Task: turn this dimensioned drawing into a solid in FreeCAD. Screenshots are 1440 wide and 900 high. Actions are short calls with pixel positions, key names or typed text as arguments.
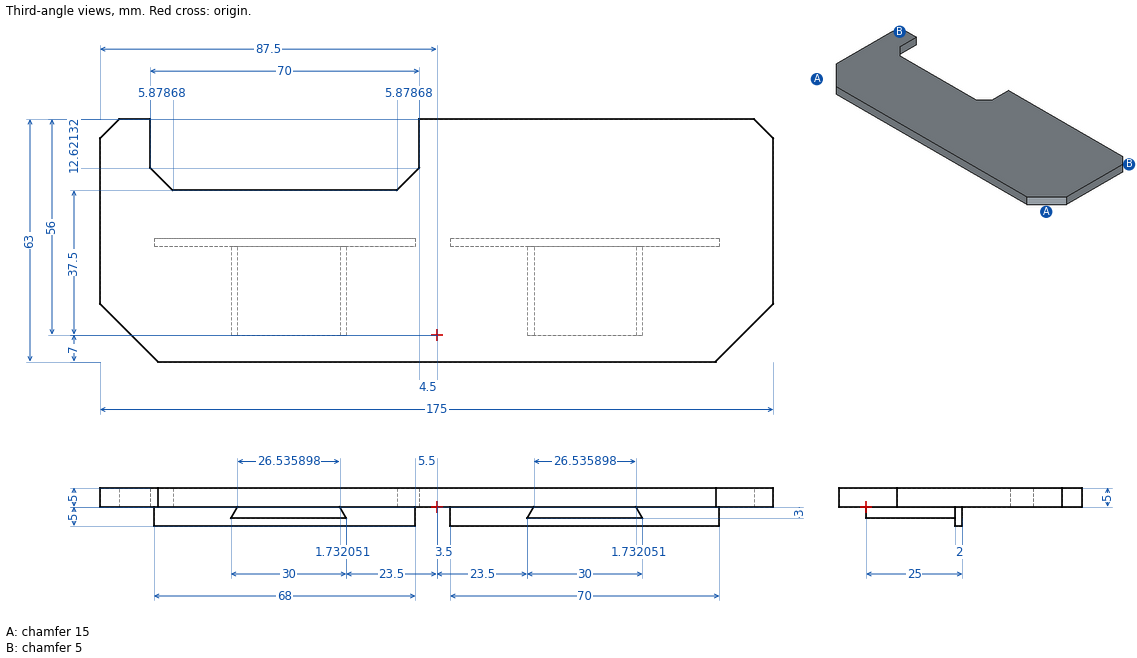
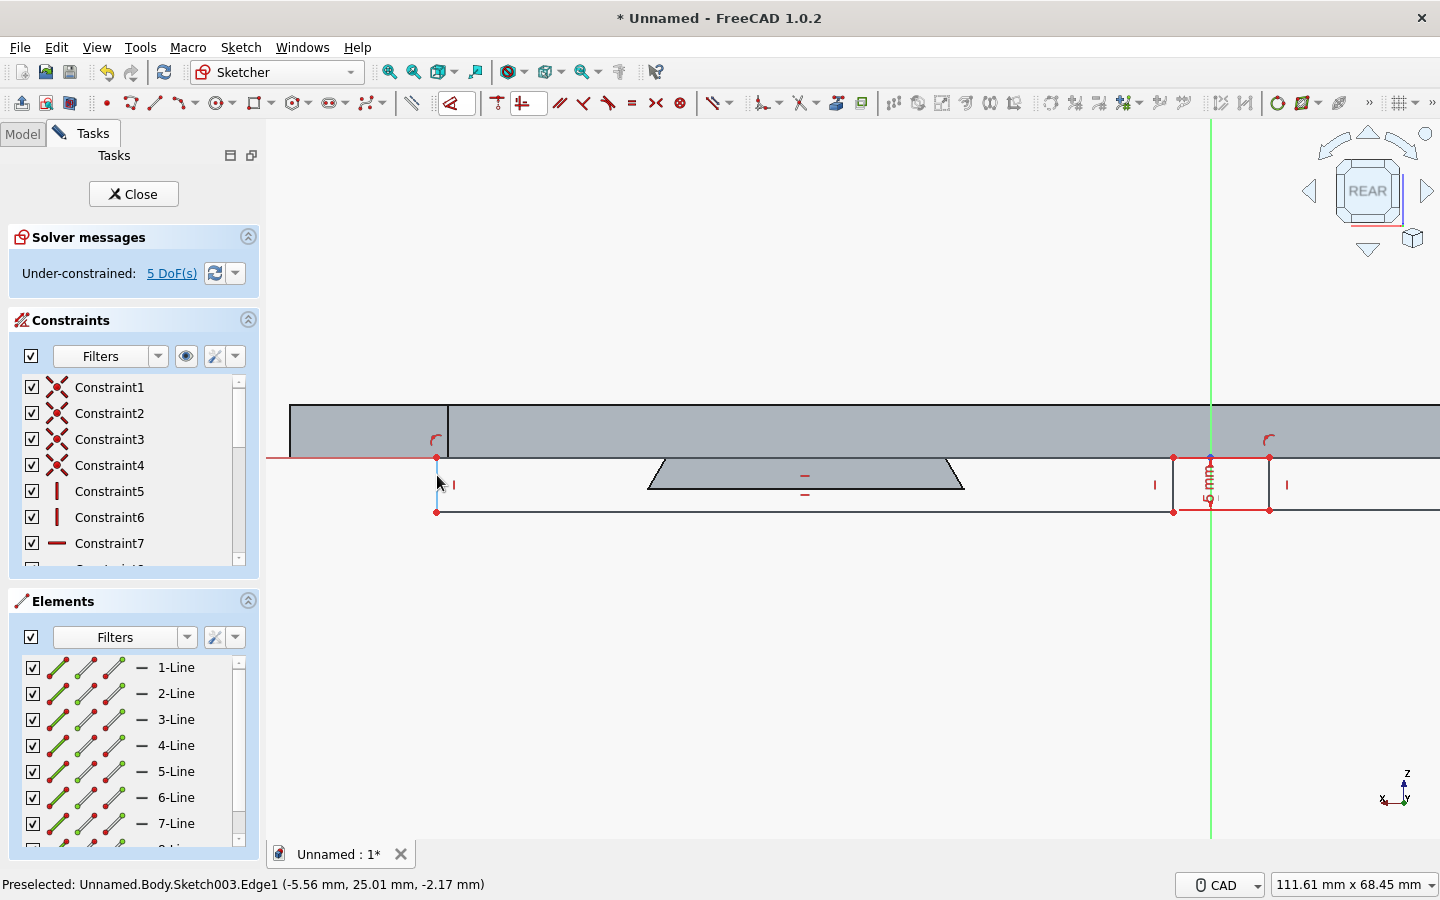
click(437, 474)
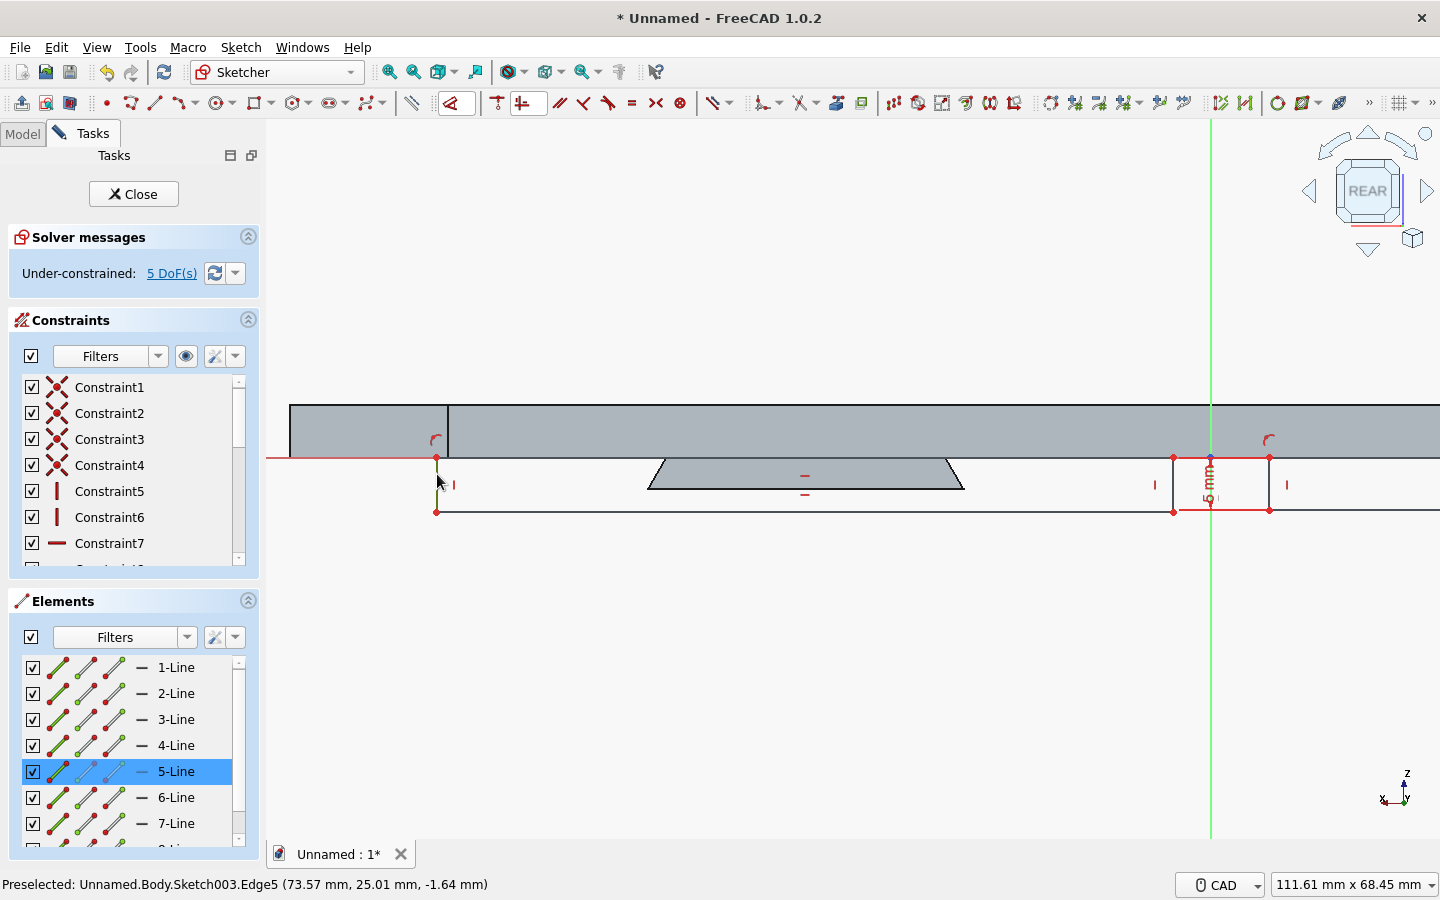
key(i)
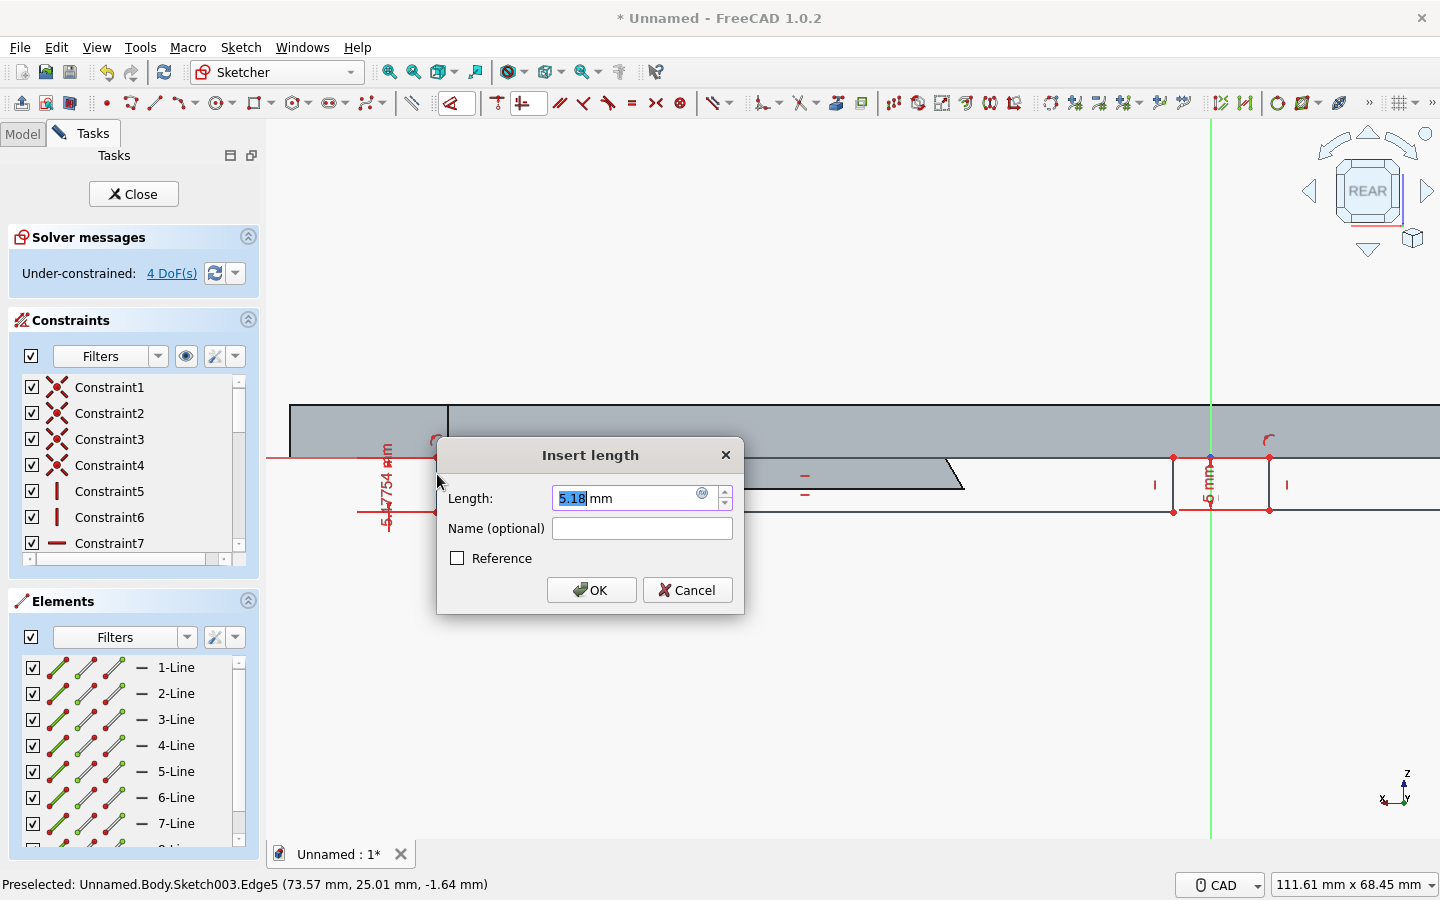
text(5)
key(Return)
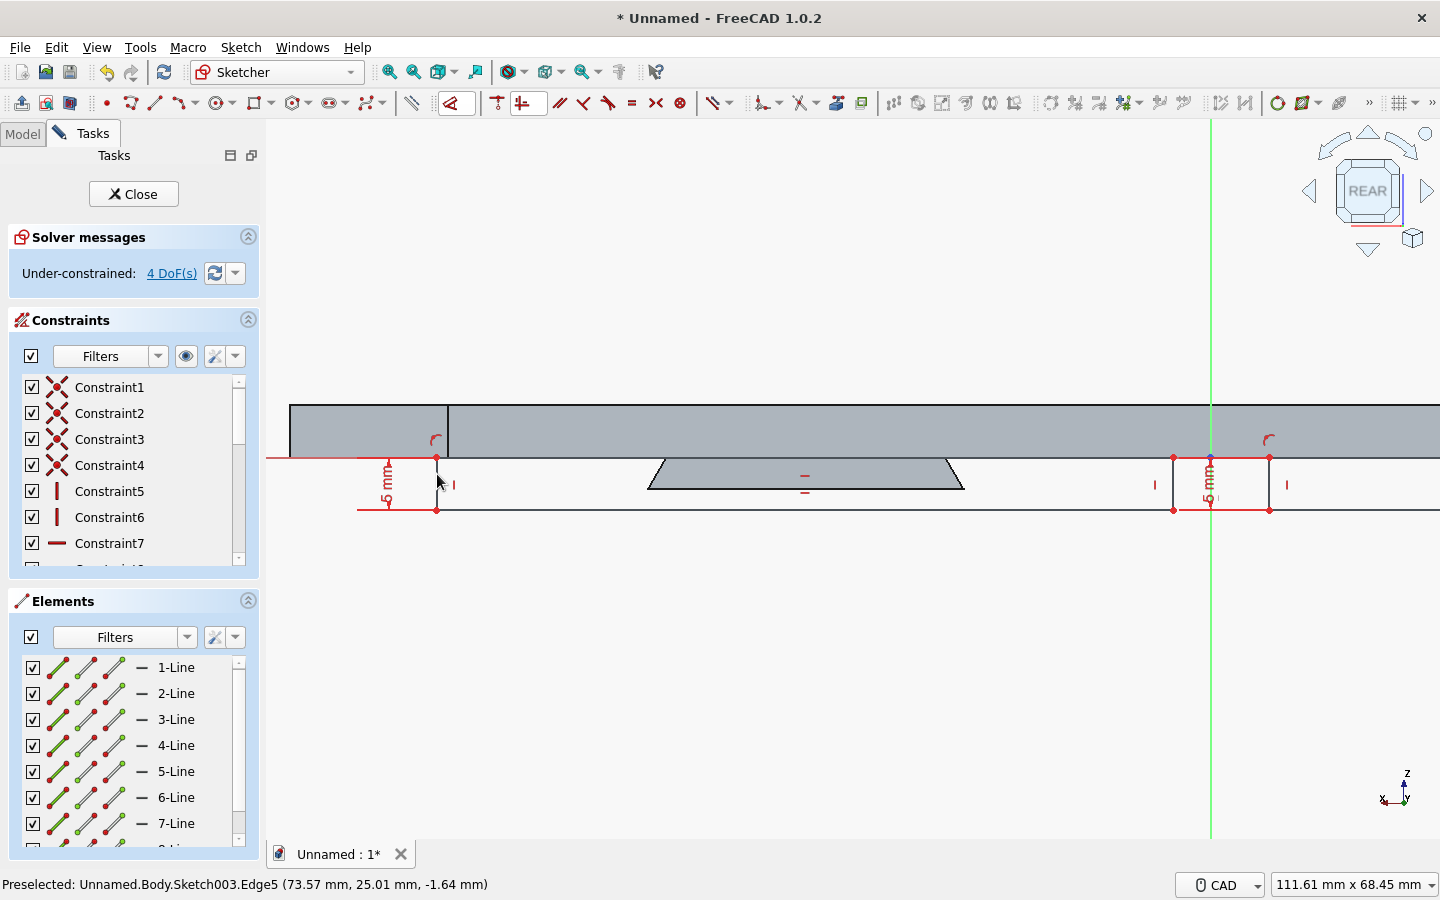
scroll(437, 475, down, 4)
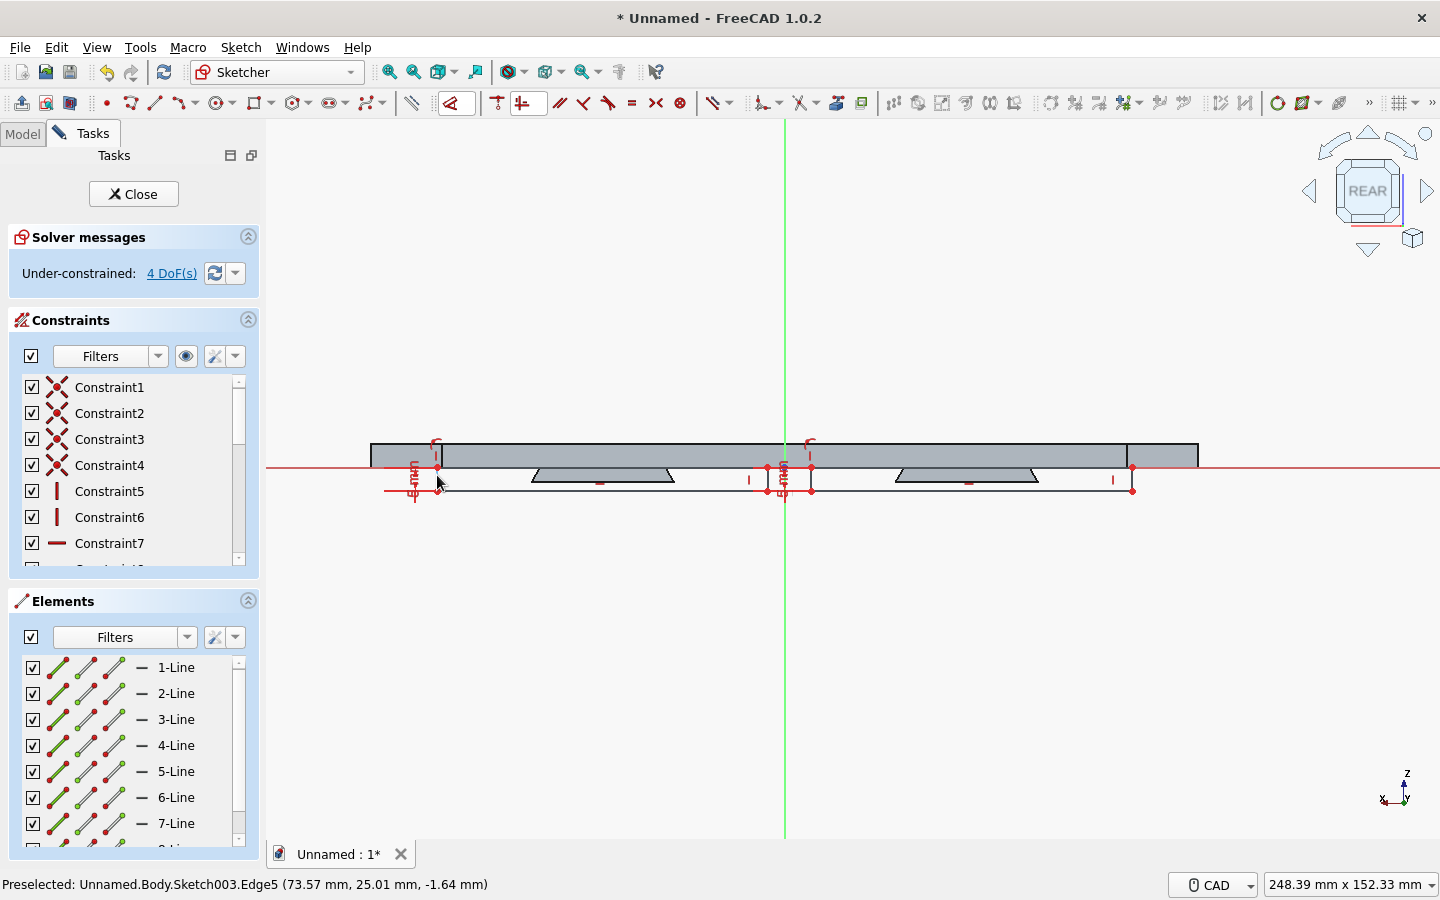
click(907, 491)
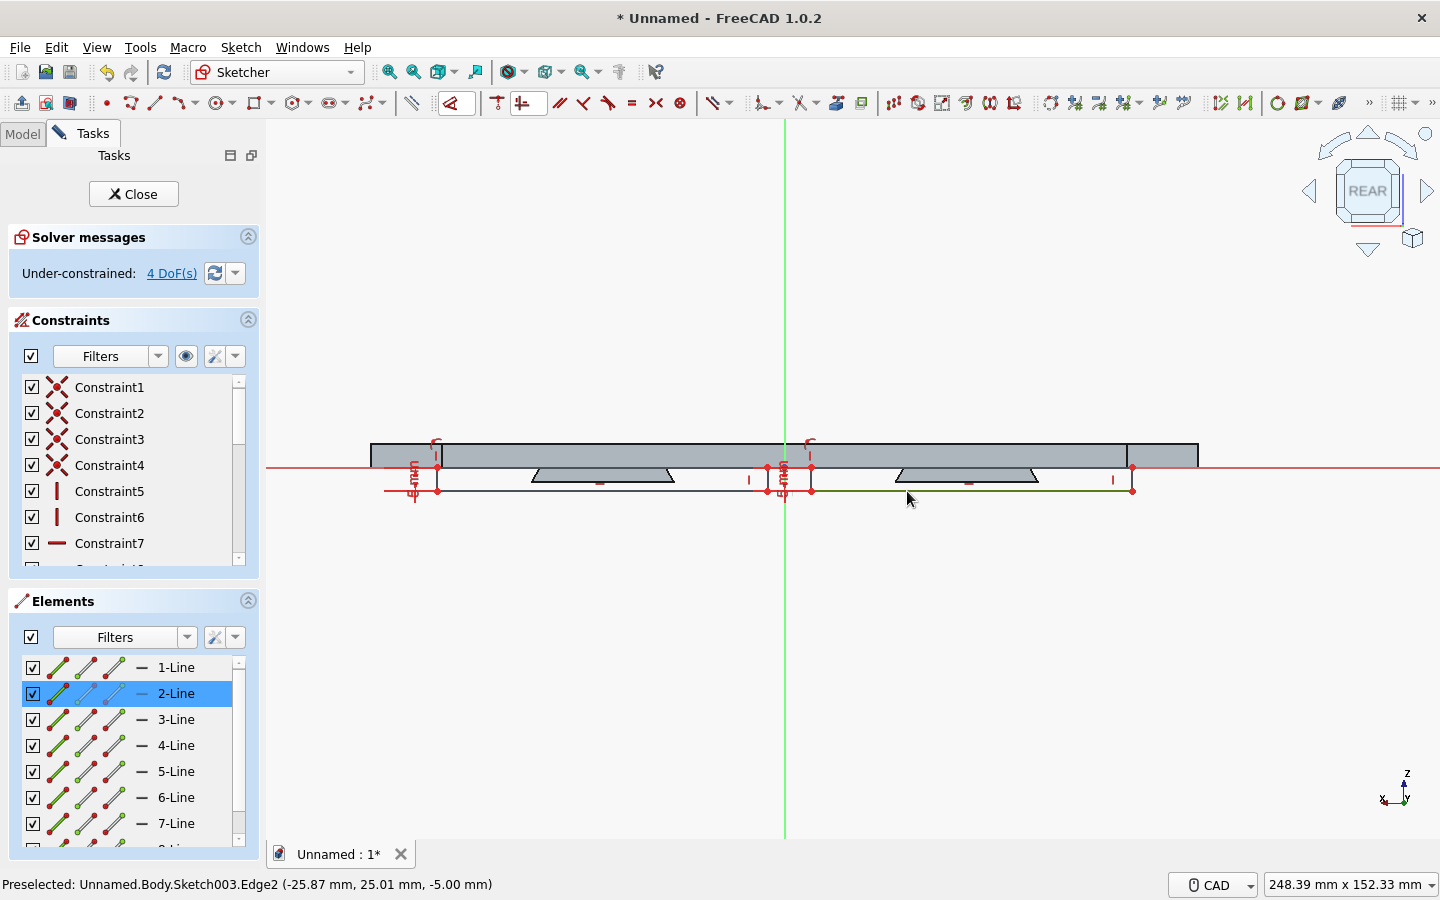
click(470, 104)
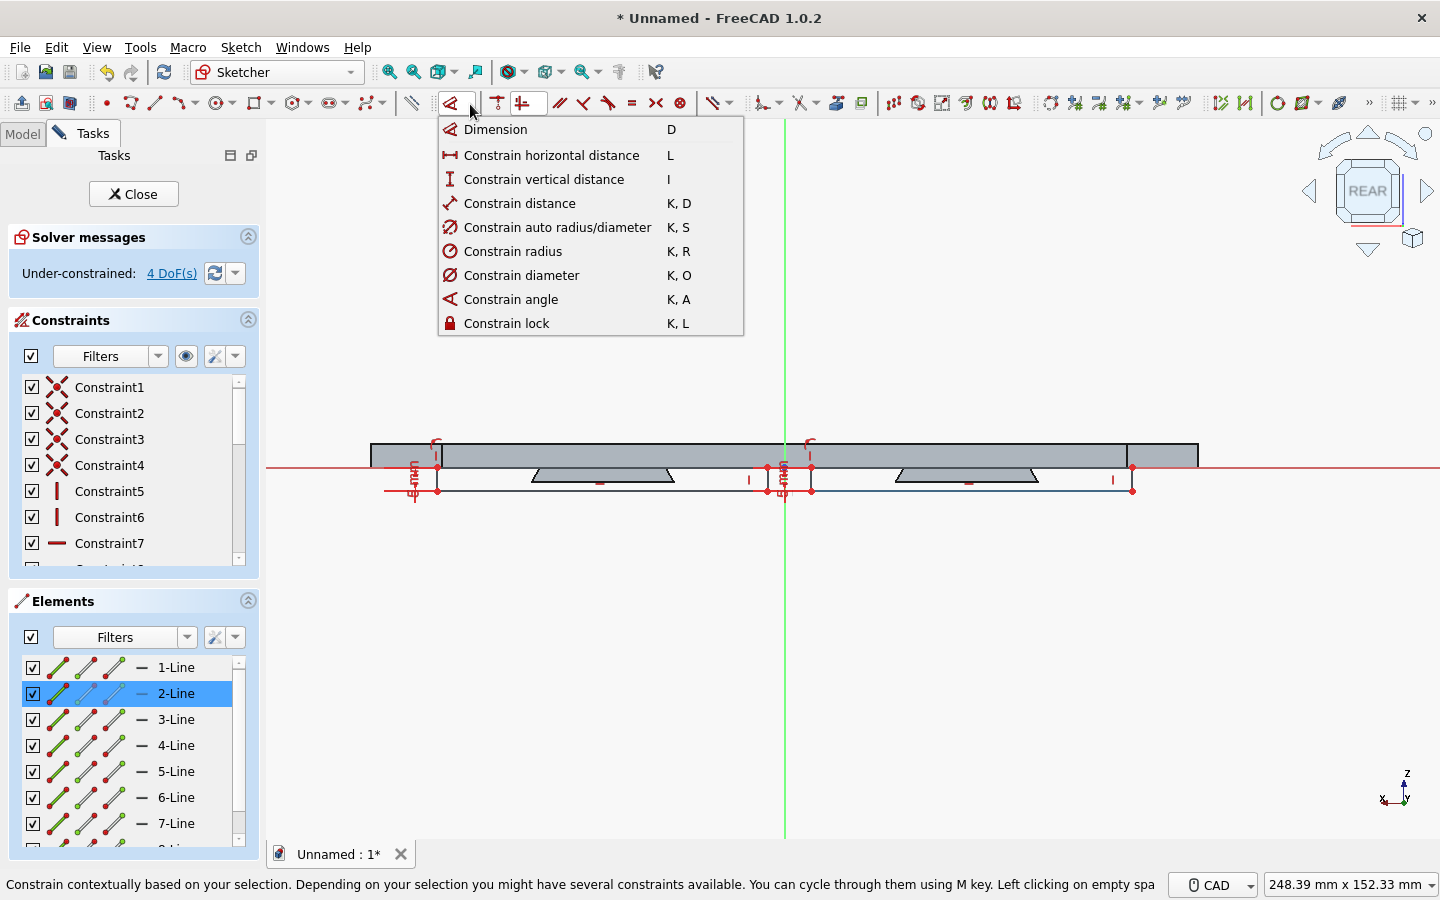
click(591, 155)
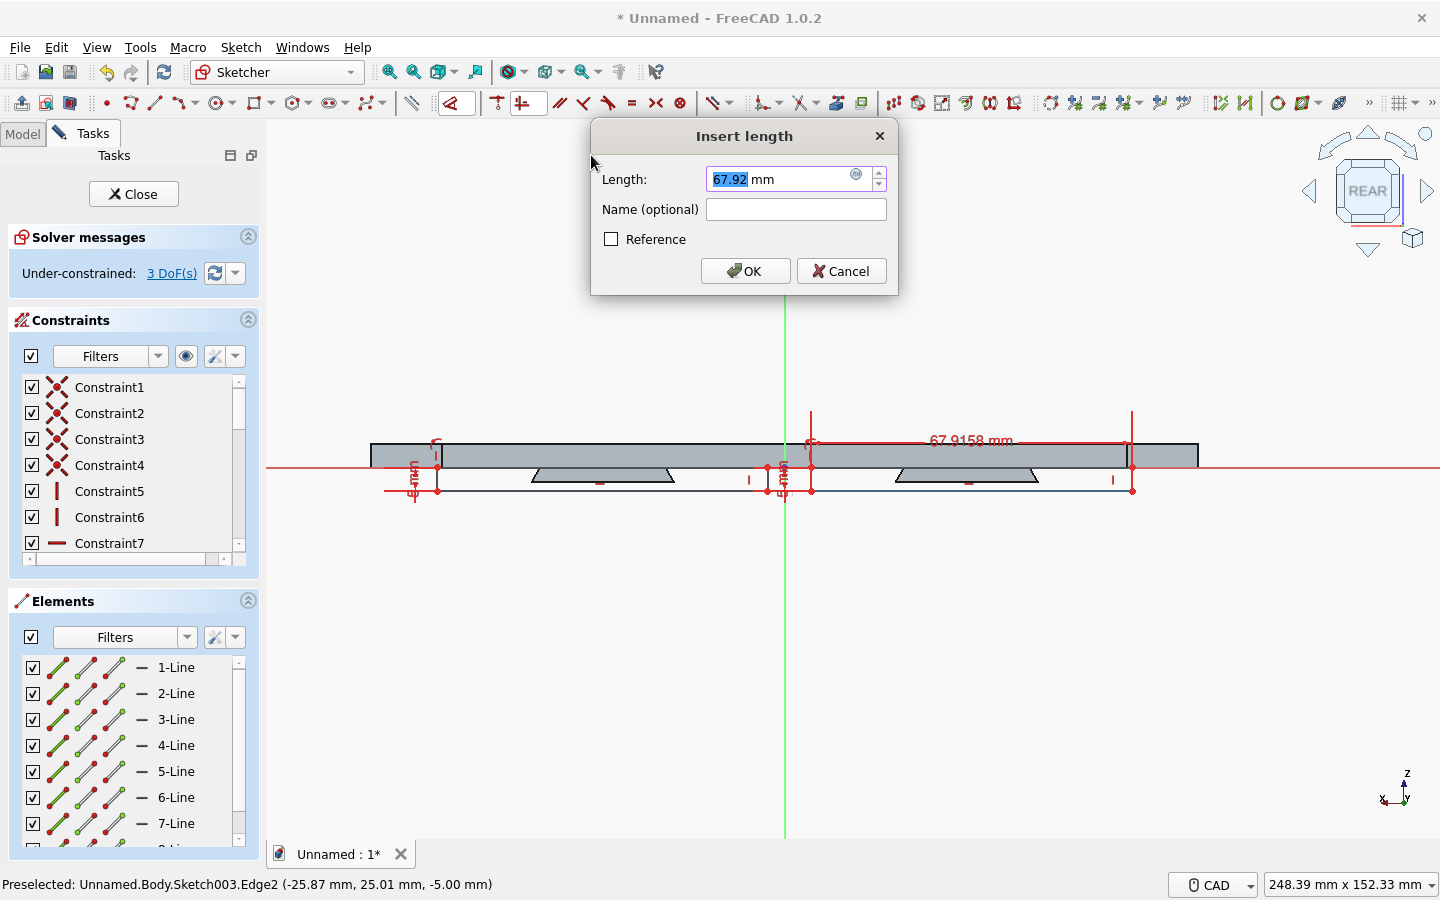
text(68)
key(Return)